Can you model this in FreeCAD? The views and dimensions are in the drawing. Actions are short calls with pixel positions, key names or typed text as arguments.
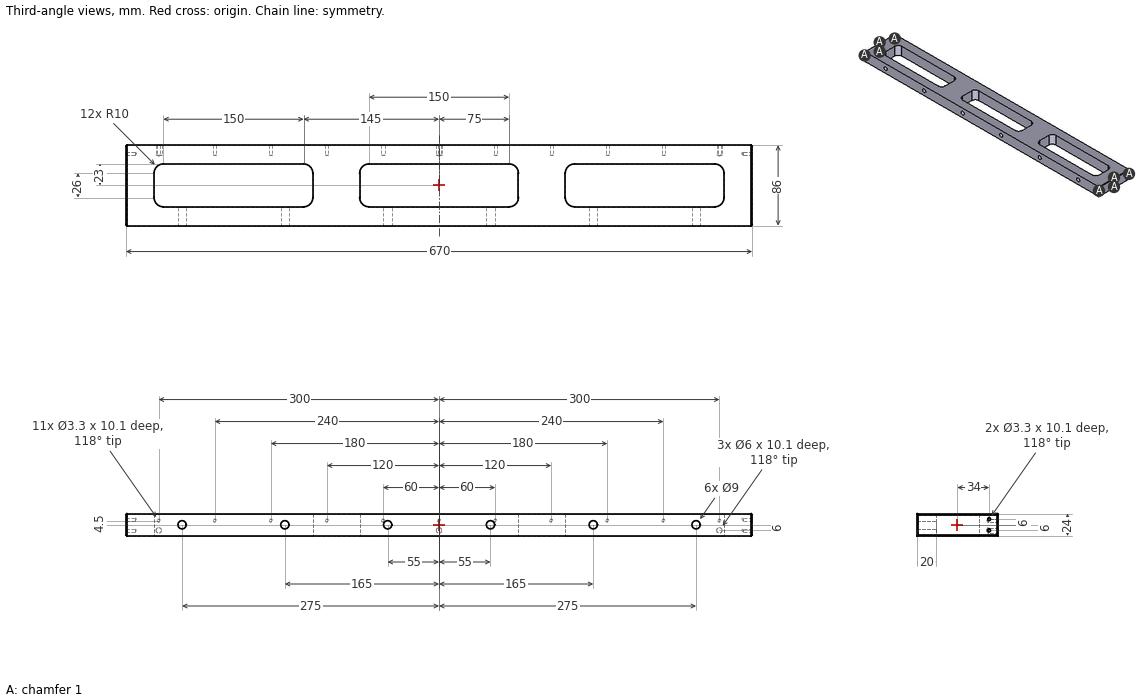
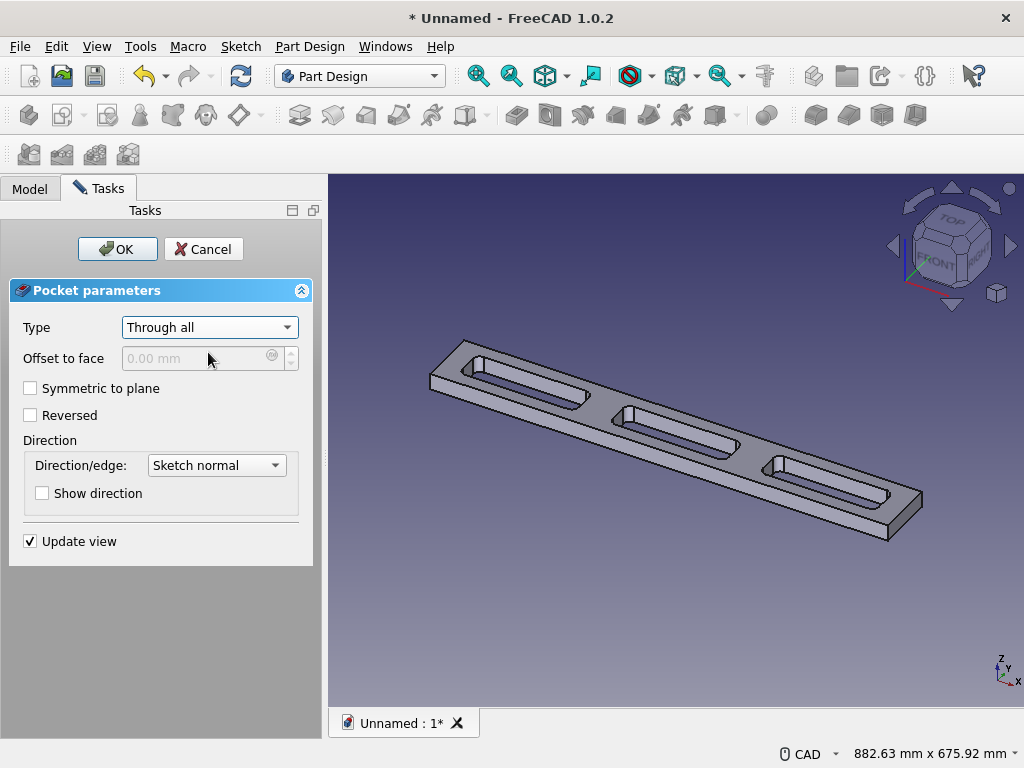
click(118, 249)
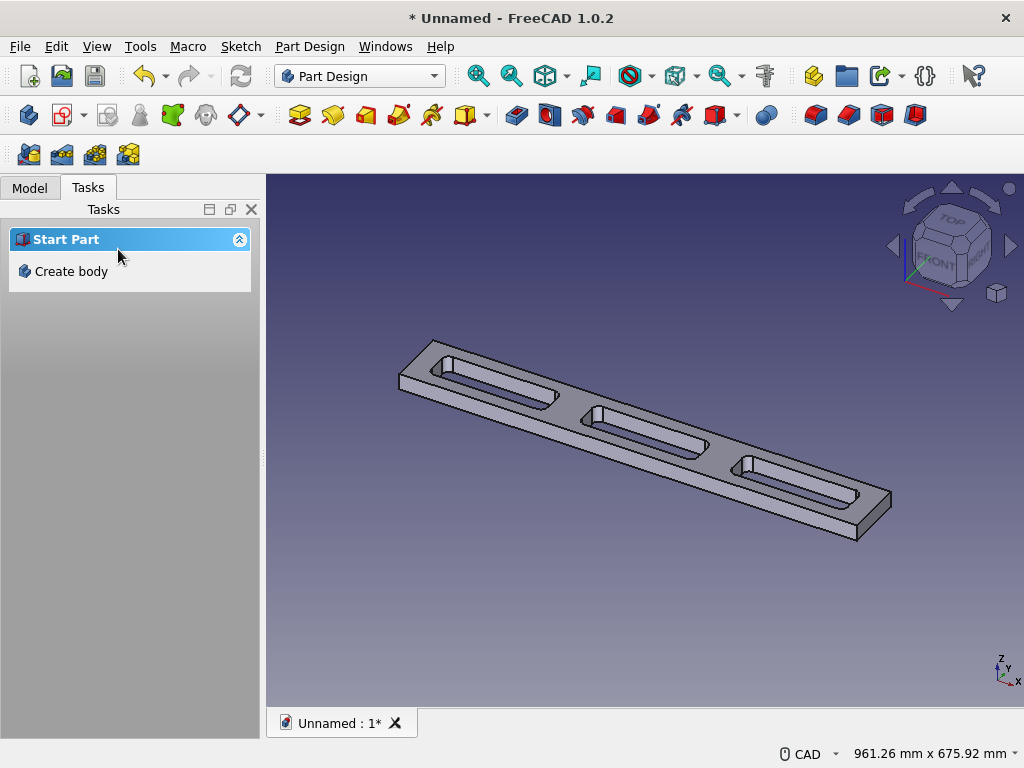
key(0)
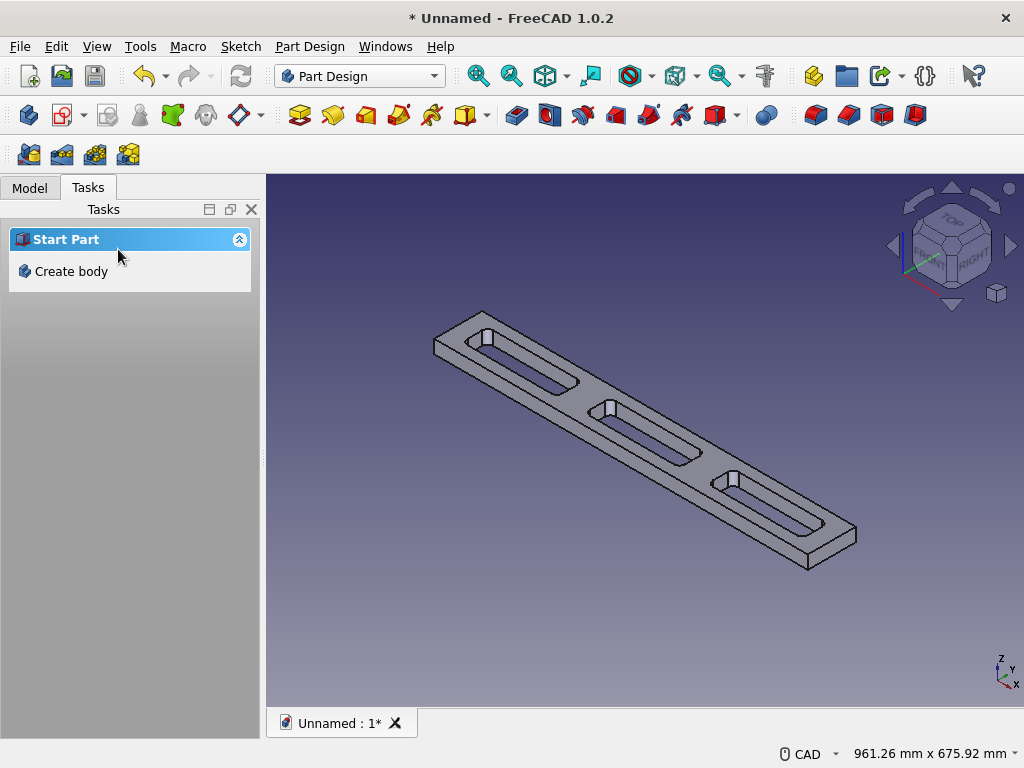
key(1)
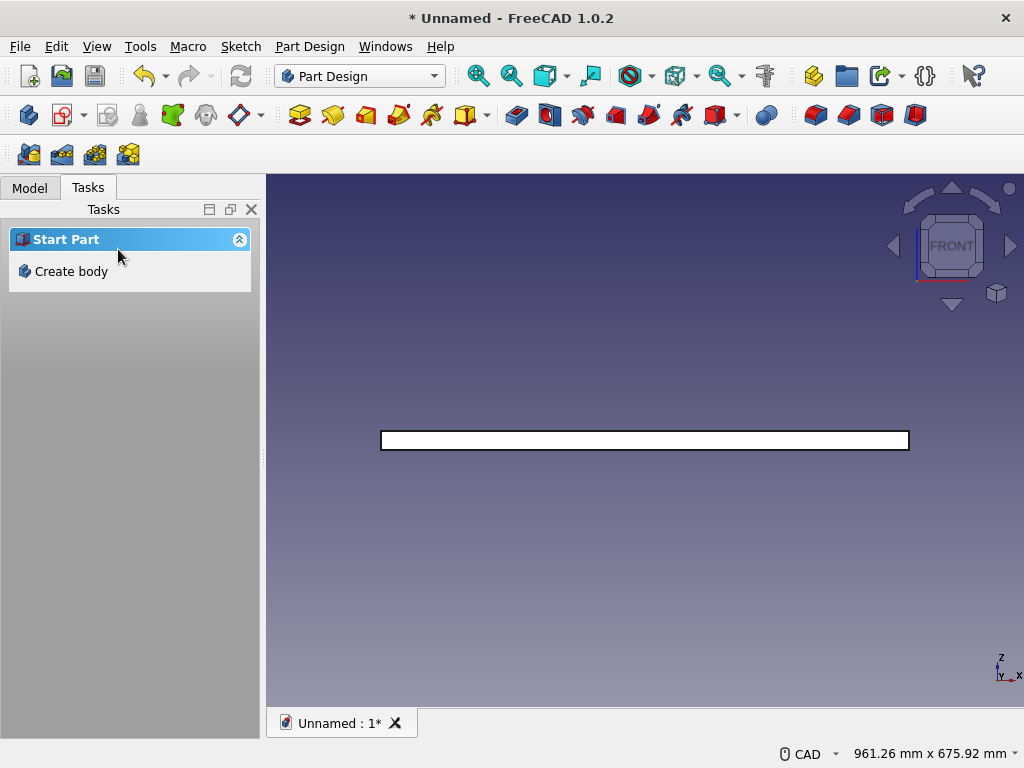
click(871, 439)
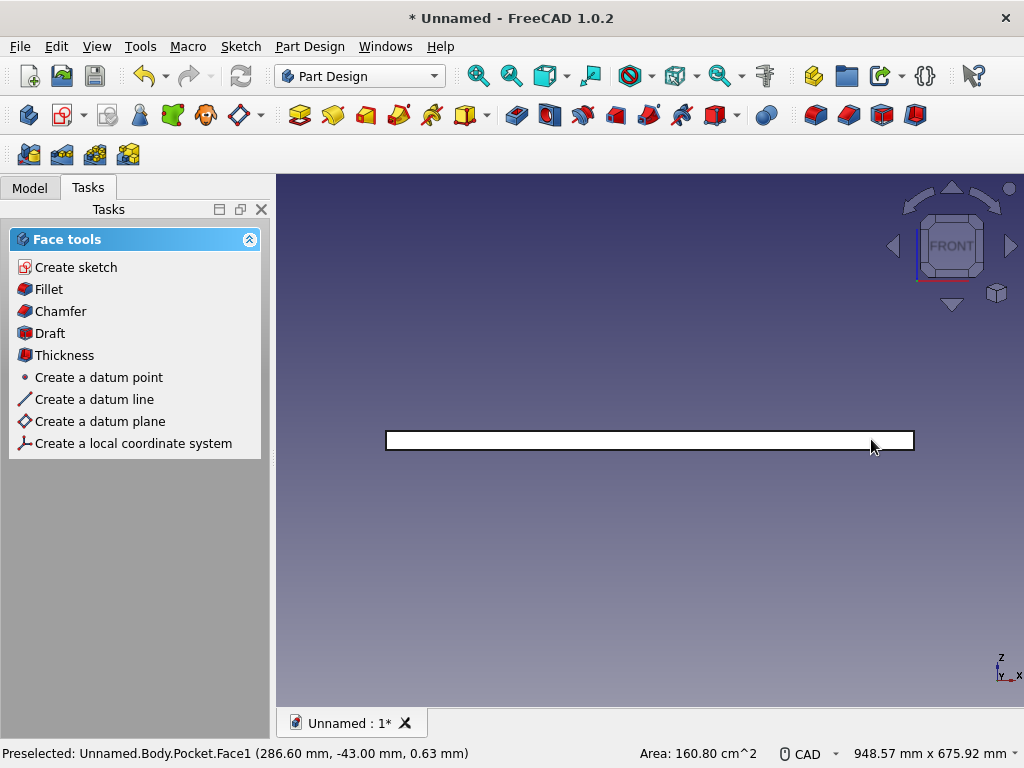
click(62, 116)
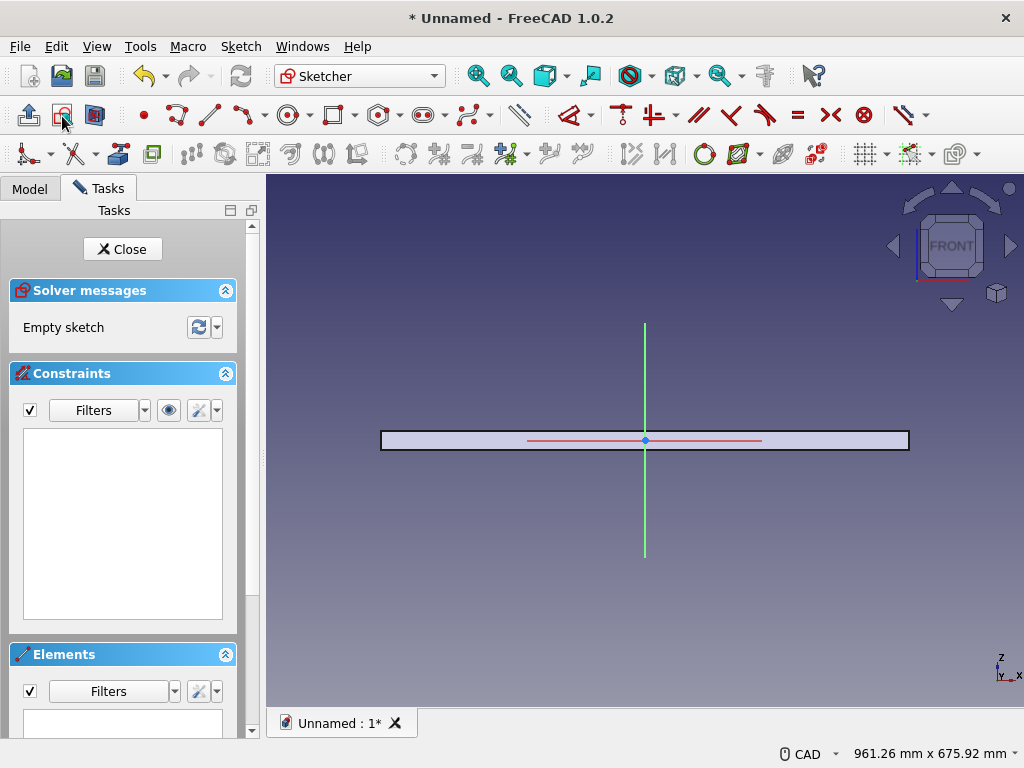
scroll(294, 441, down, 1)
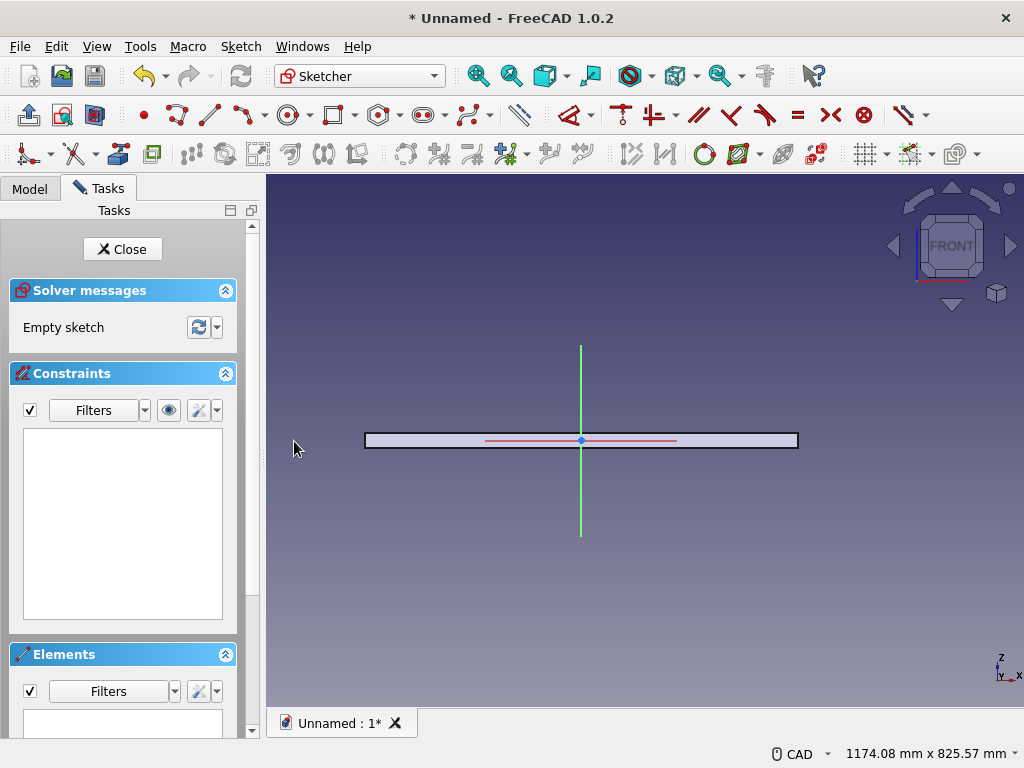
key(g)
key(c)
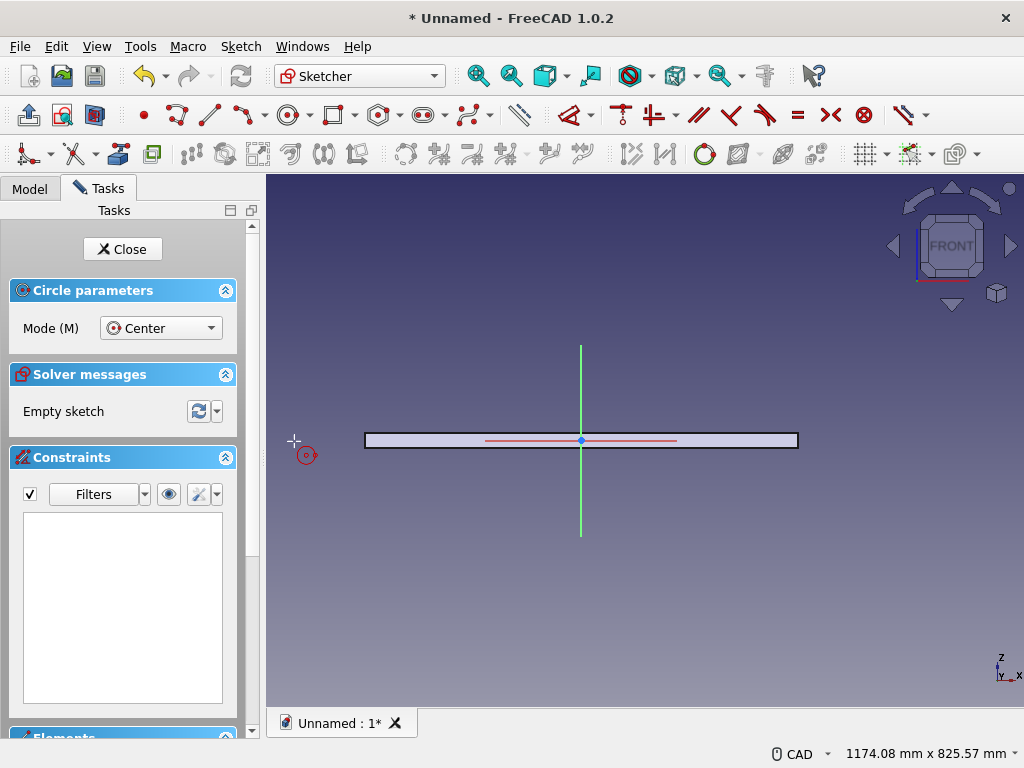
scroll(759, 441, up, 11)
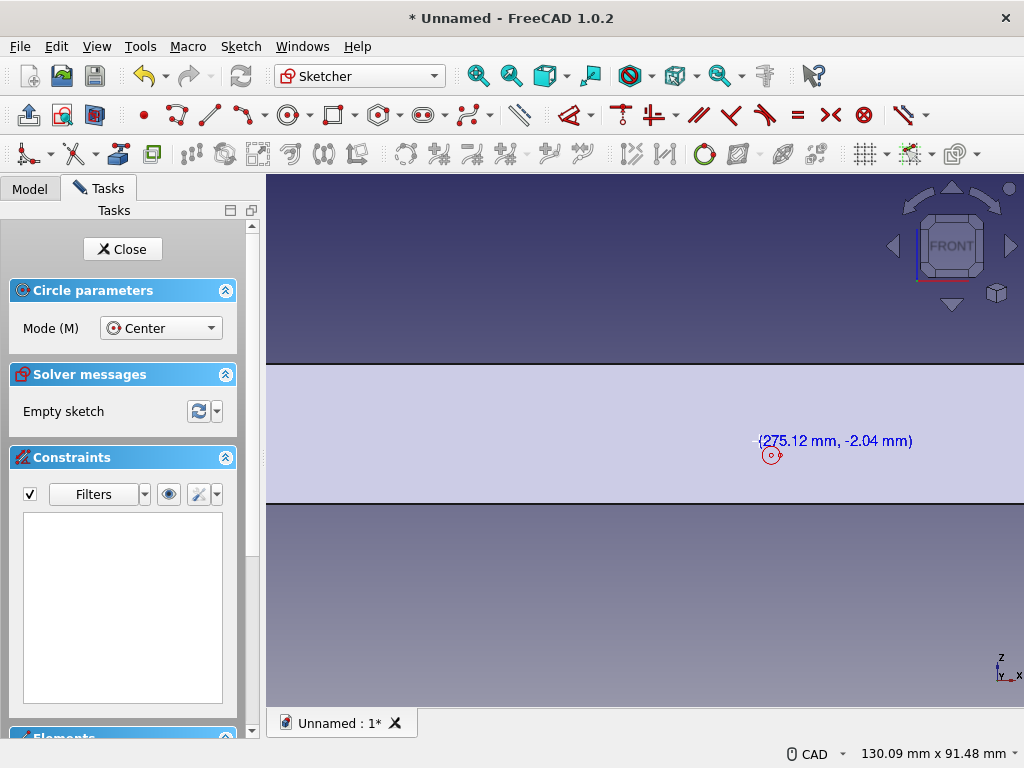
scroll(754, 441, down, 11)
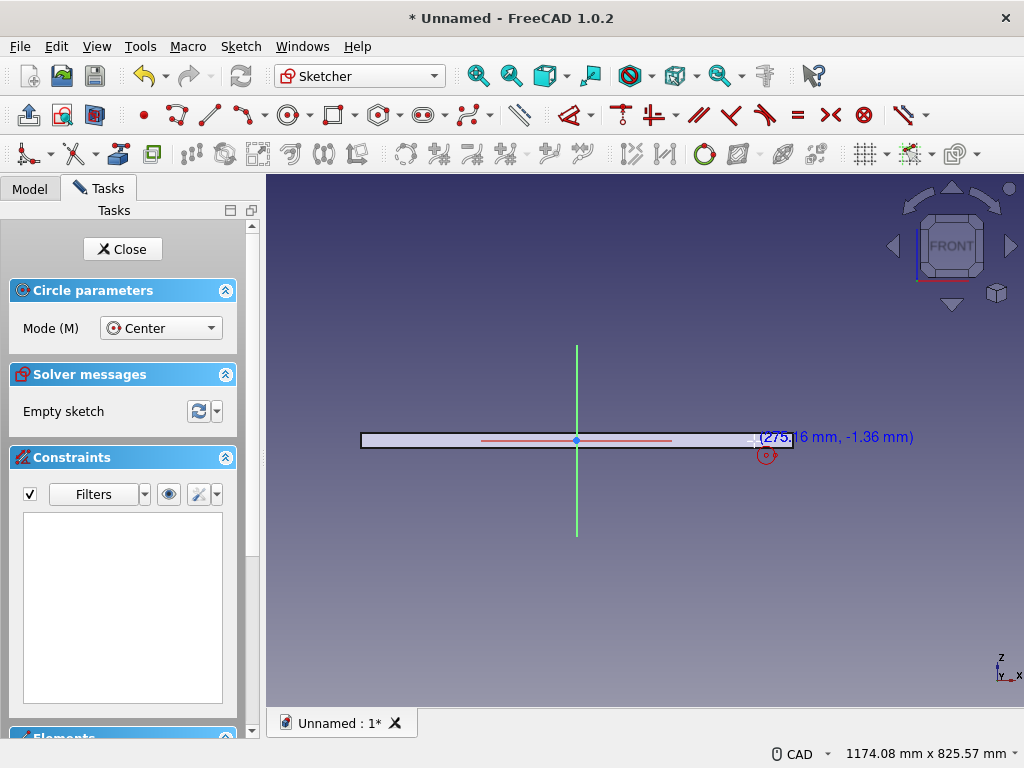
click(754, 441)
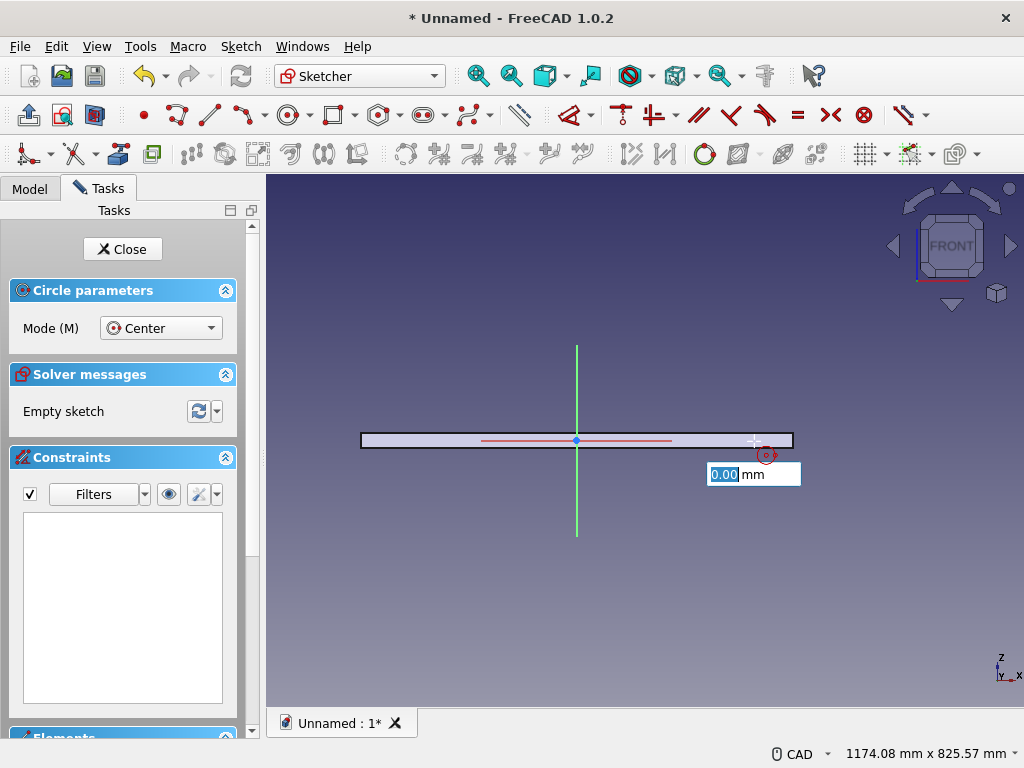
scroll(753, 443, up, 9)
move(753, 443)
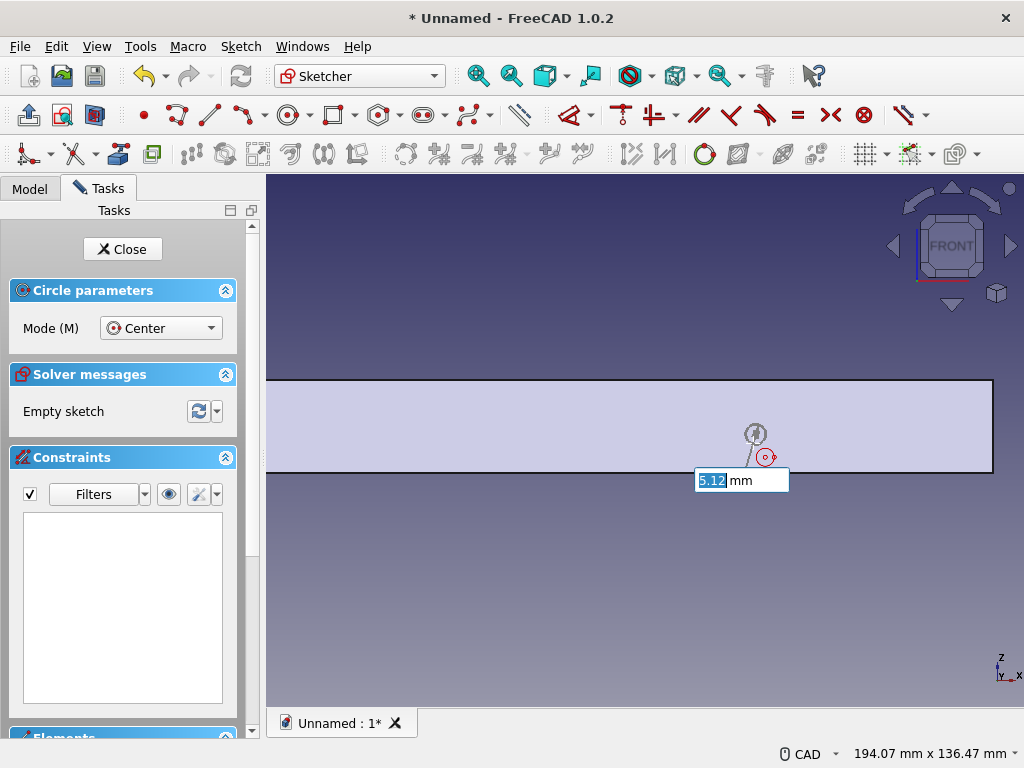
text(9)
key(Return)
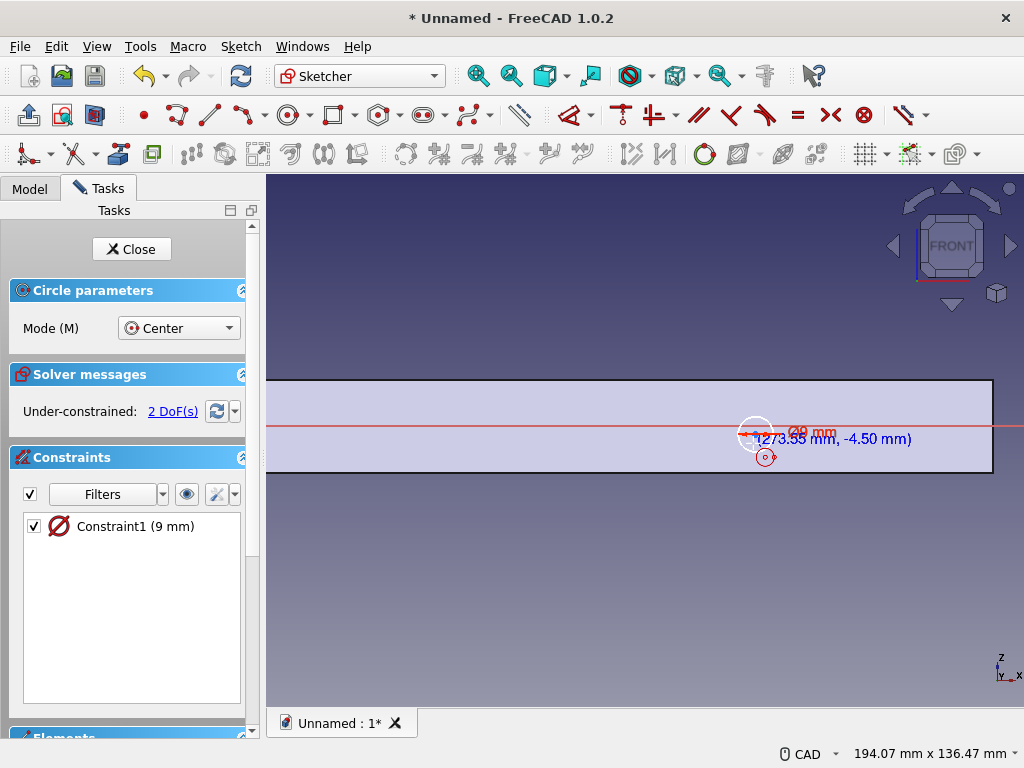
scroll(753, 443, down, 9)